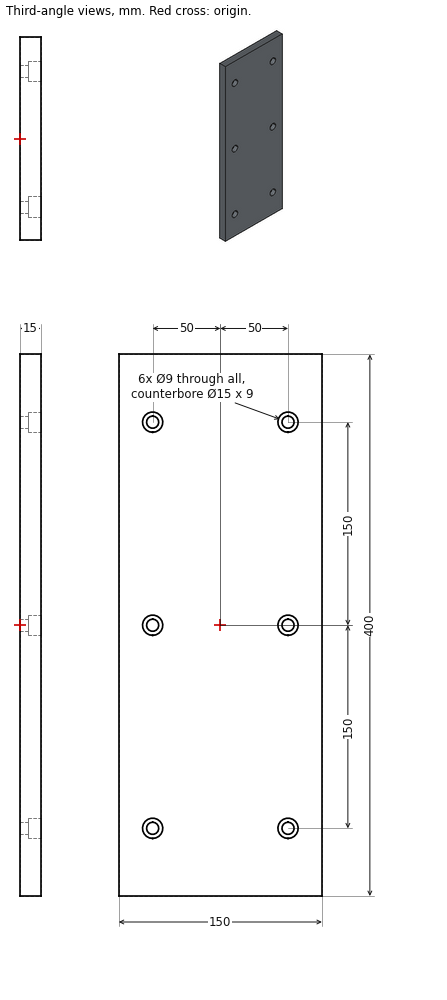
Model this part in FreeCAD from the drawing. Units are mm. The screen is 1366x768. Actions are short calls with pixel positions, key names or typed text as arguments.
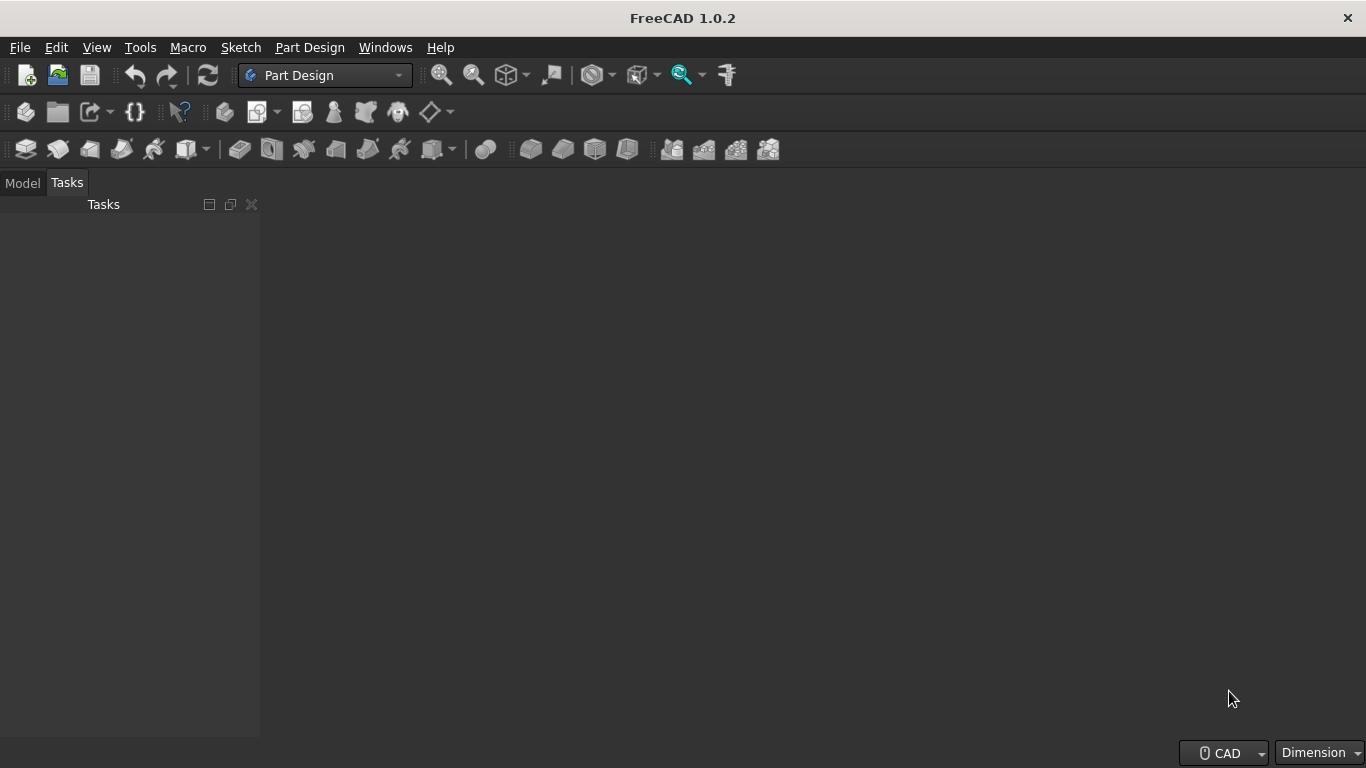
key(ctrl+n)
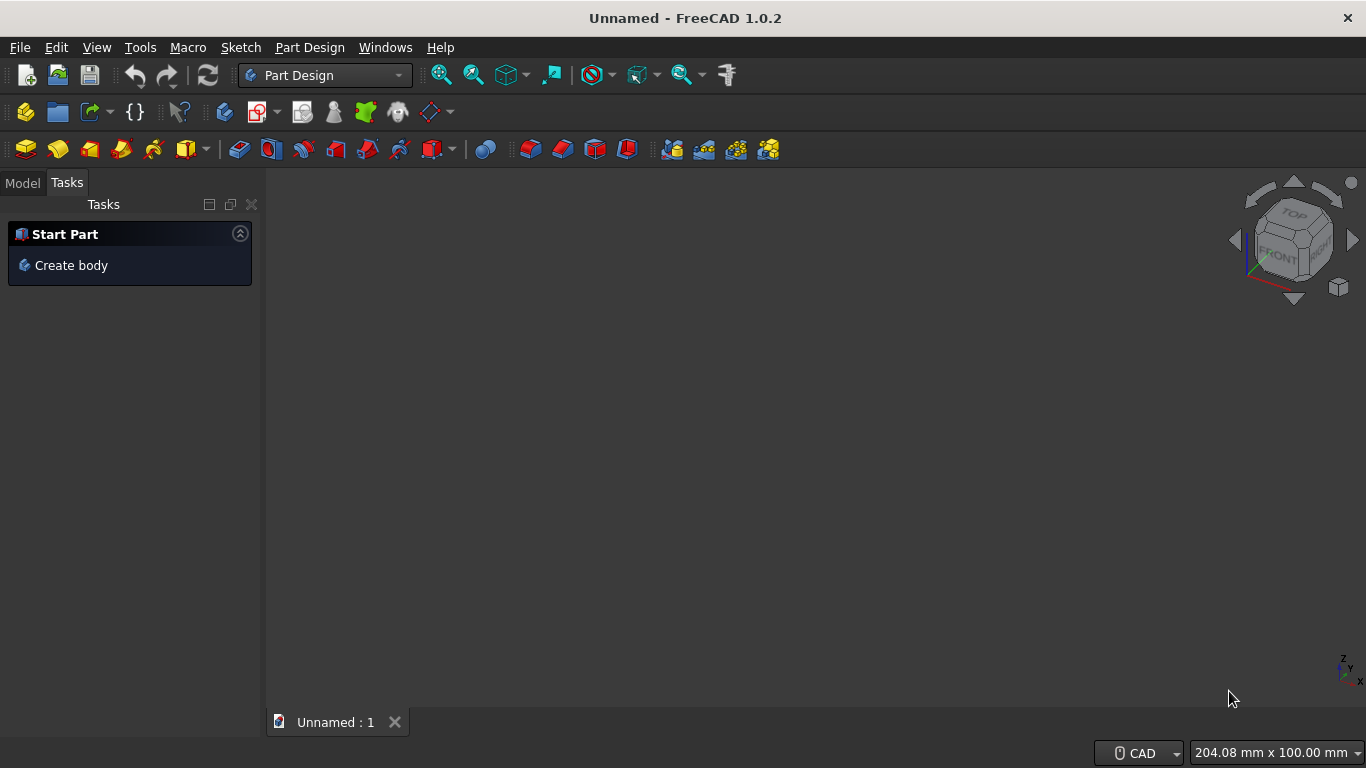
click(258, 112)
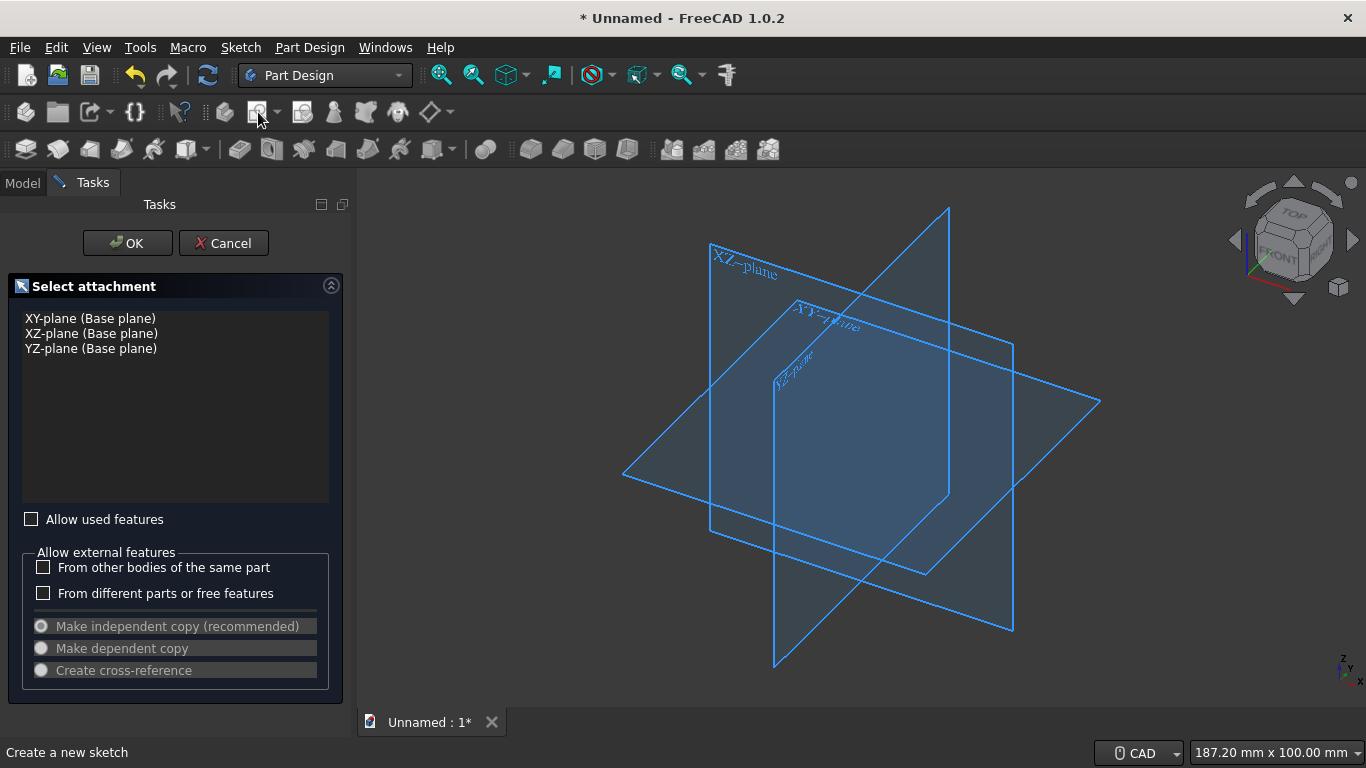
click(82, 348)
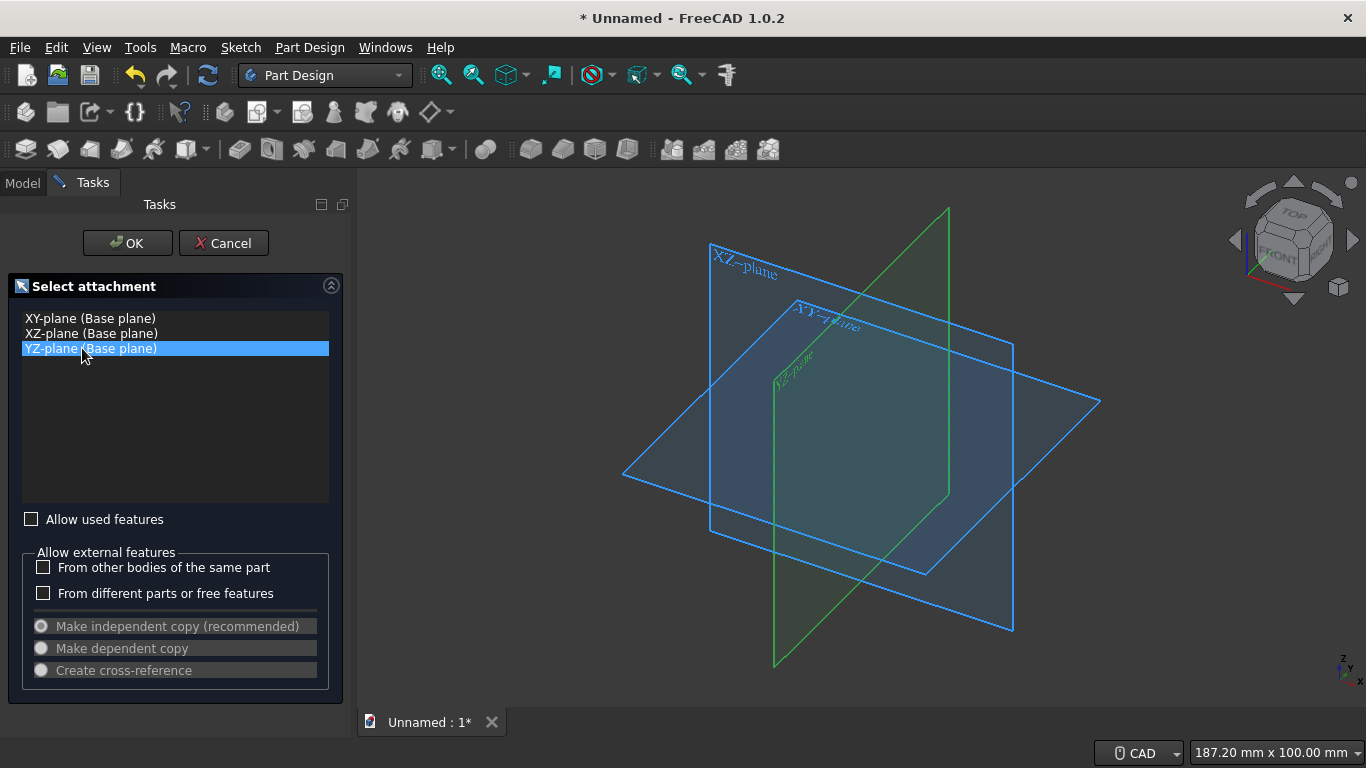
click(128, 243)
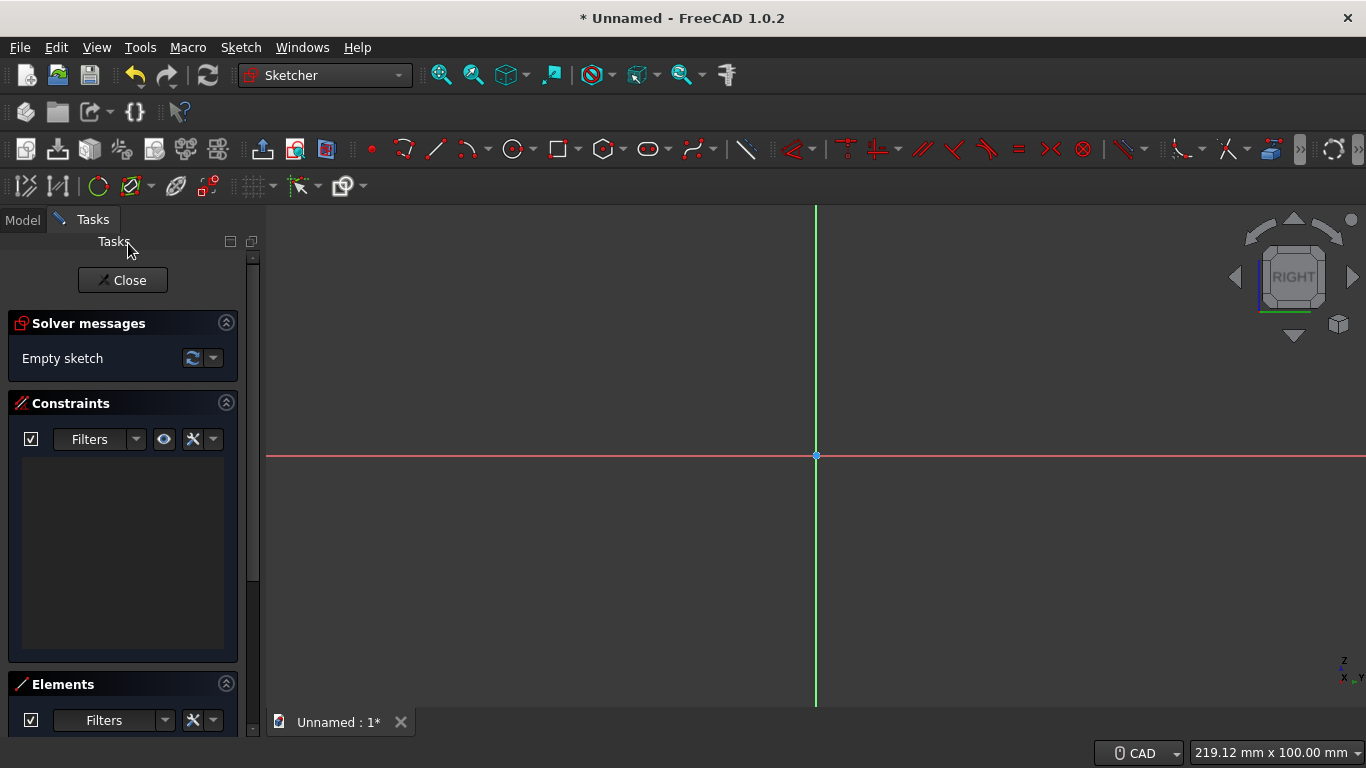
scroll(734, 456, down, 9)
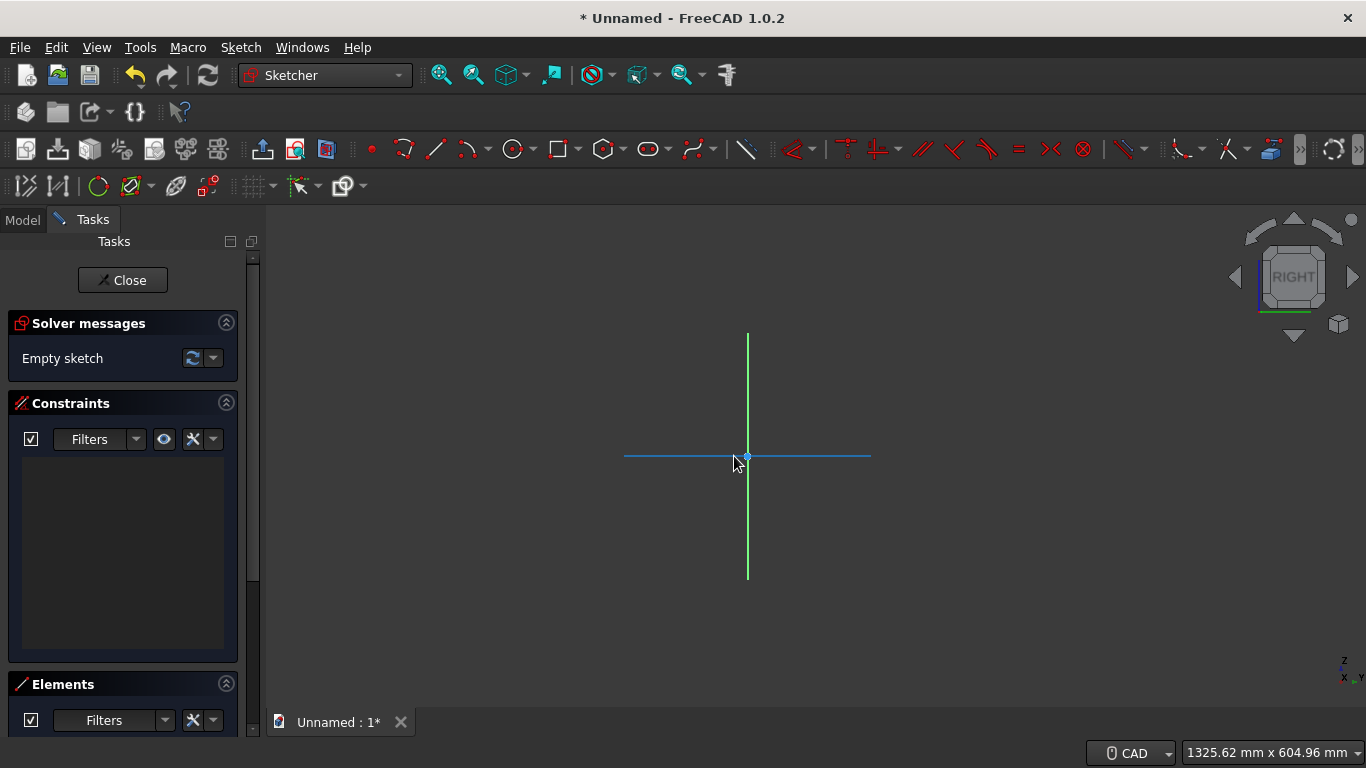
click(580, 150)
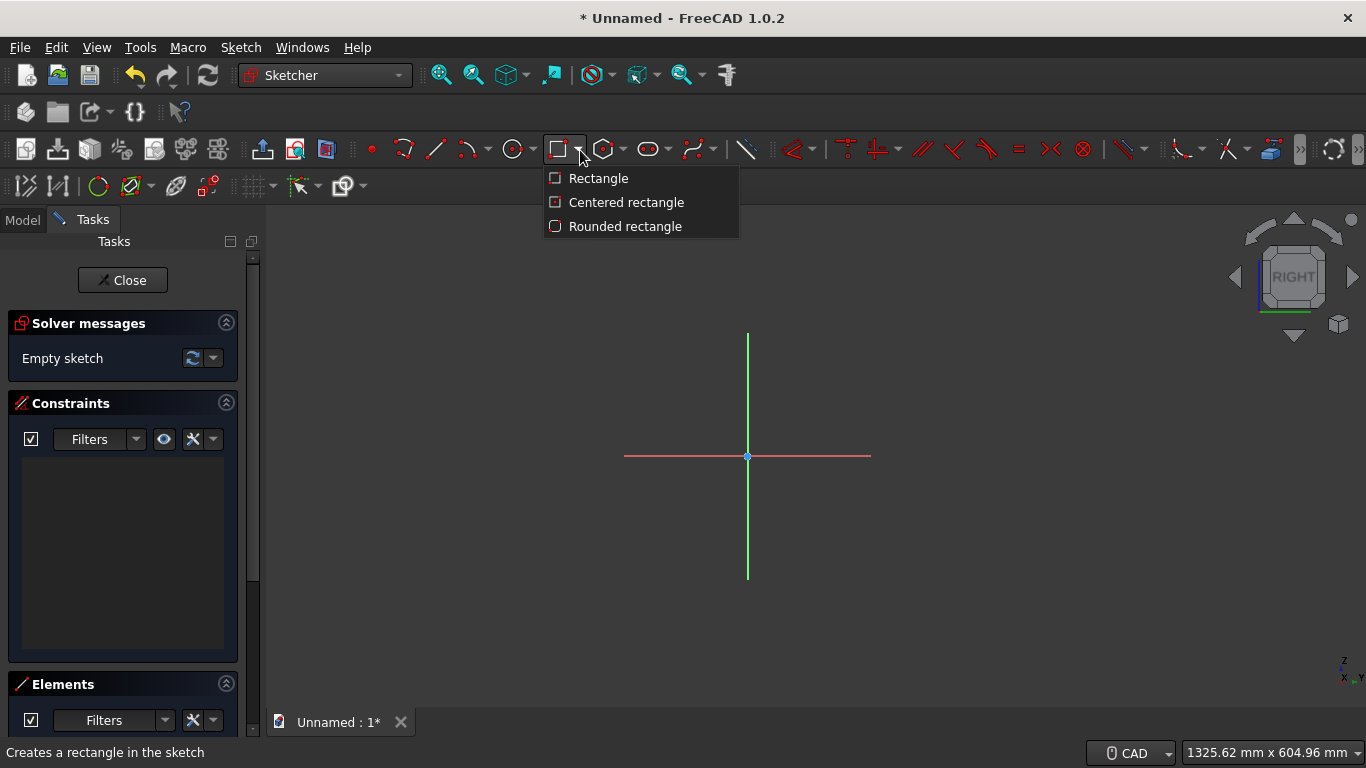
click(642, 202)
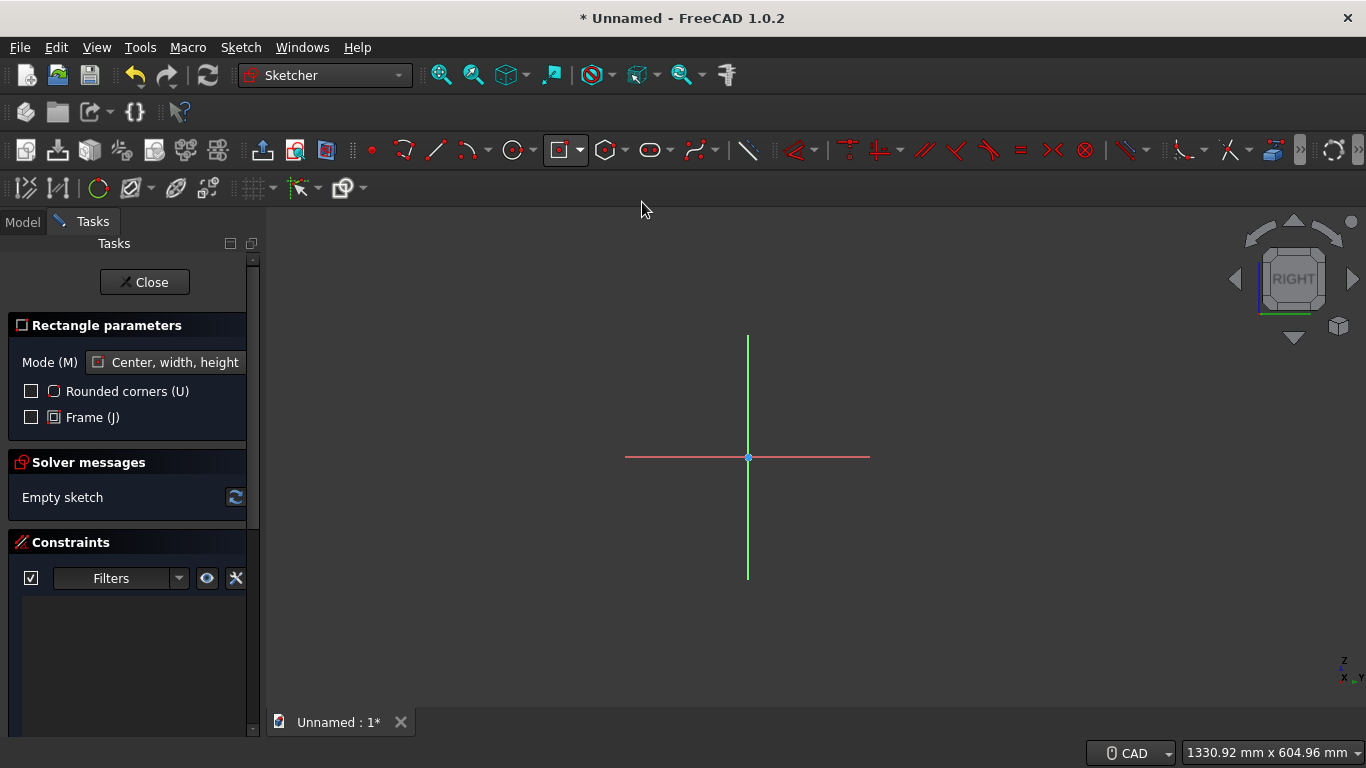
click(748, 457)
click(810, 292)
key(Escape)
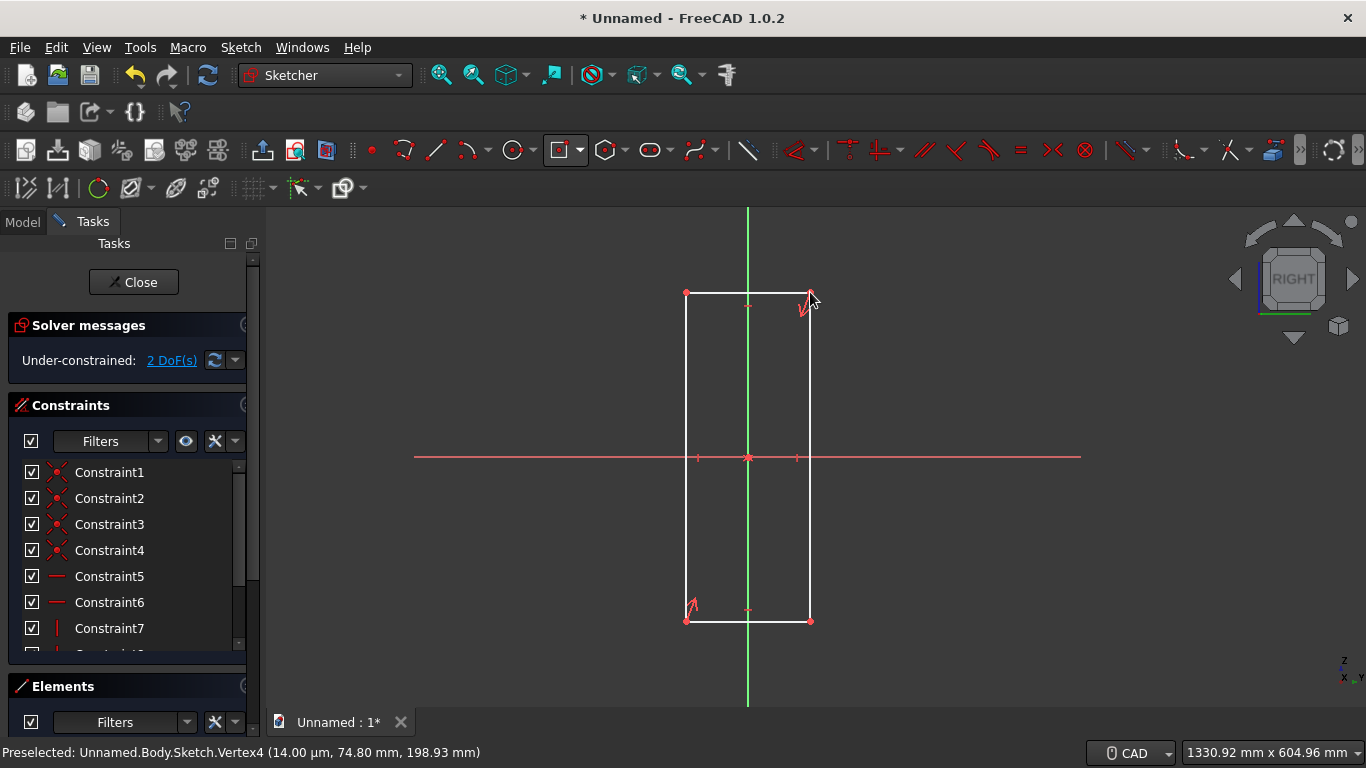
key(d)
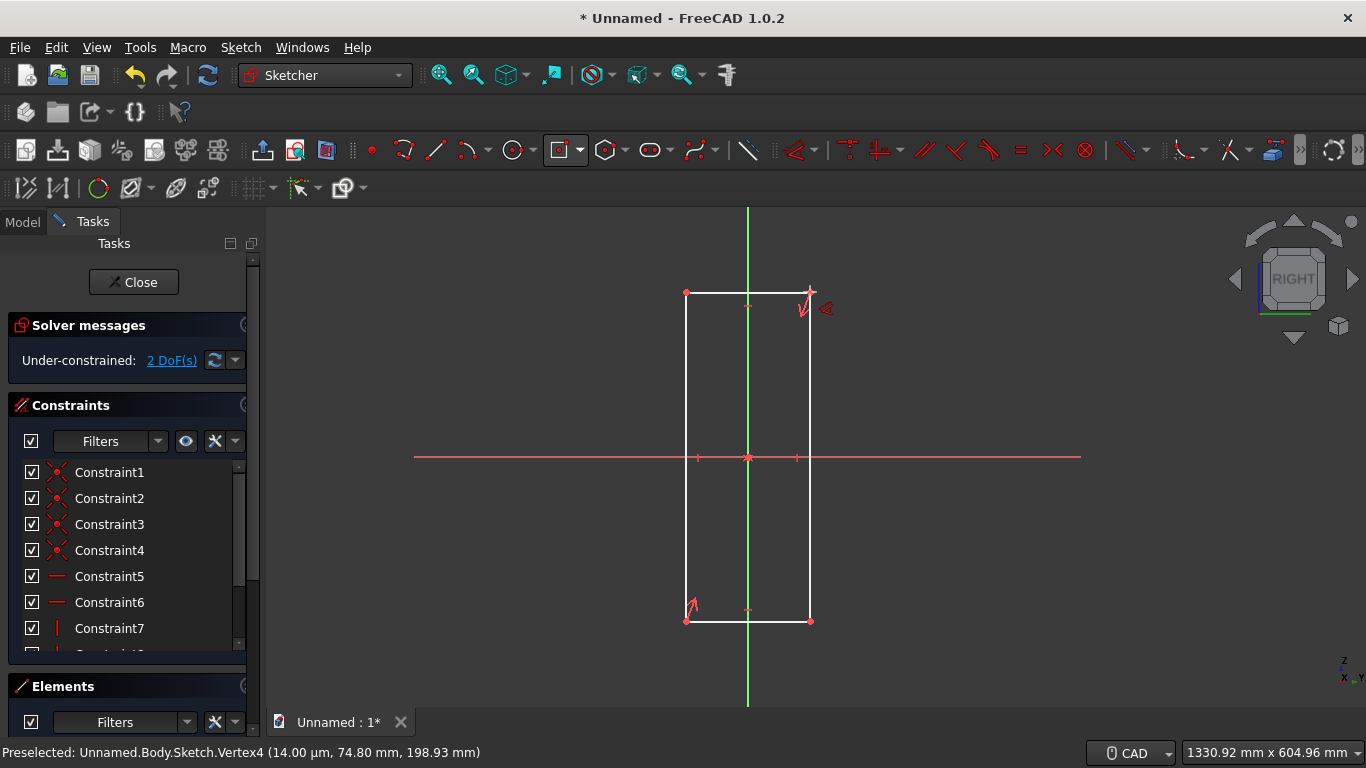
click(723, 622)
click(720, 656)